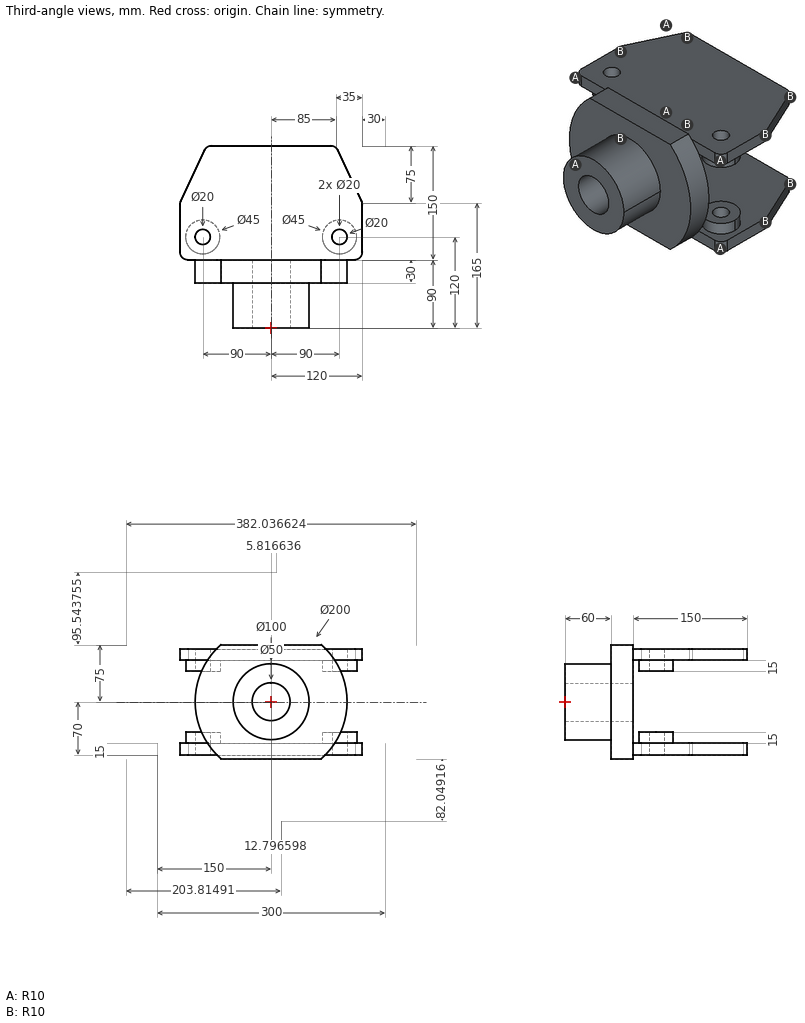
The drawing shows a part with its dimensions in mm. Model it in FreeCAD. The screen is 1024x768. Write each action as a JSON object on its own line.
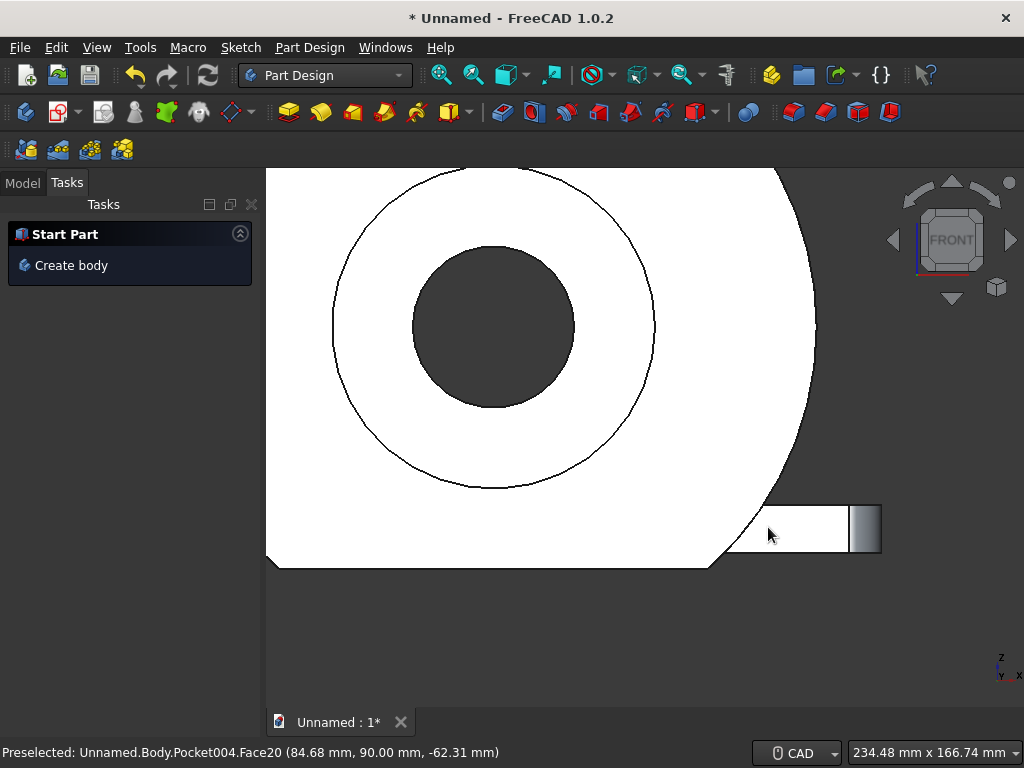
{"action": "left_click", "coordinate": [442, 76]}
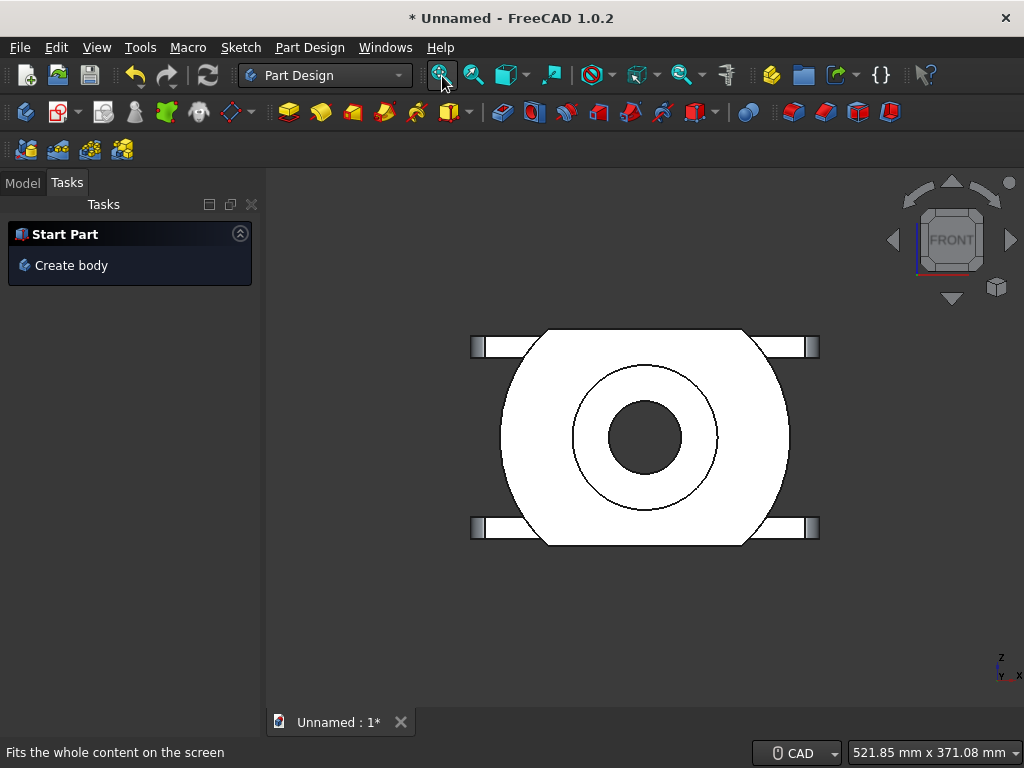
{"action": "key", "text": "3"}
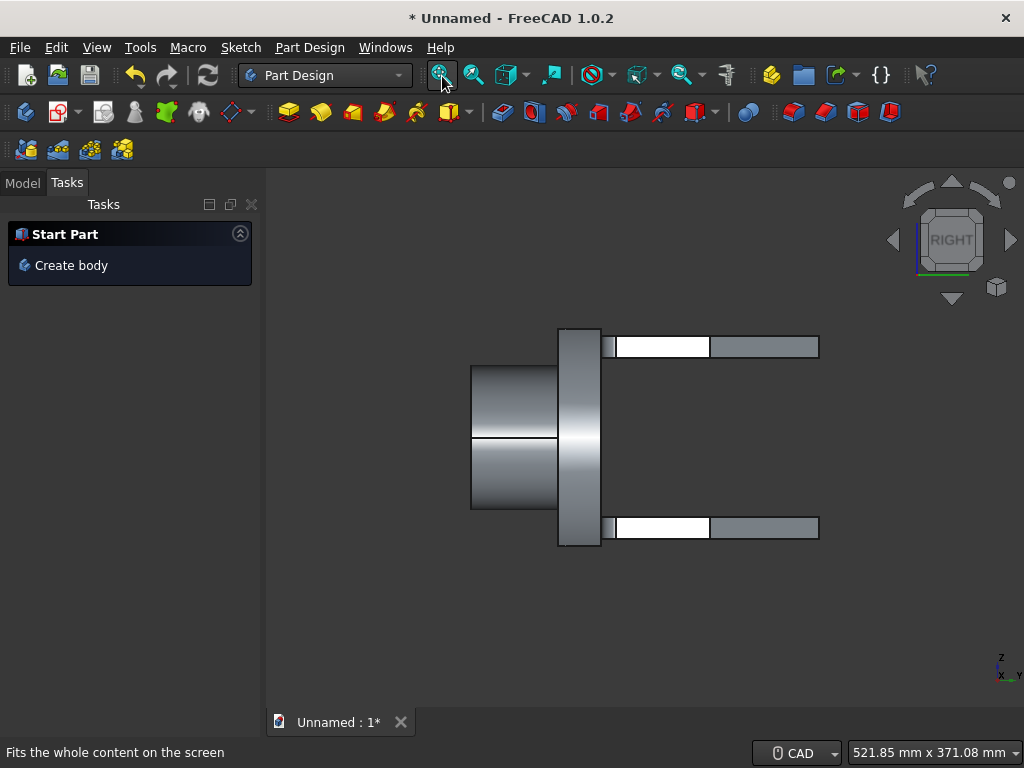
{"action": "left_click", "coordinate": [710, 346]}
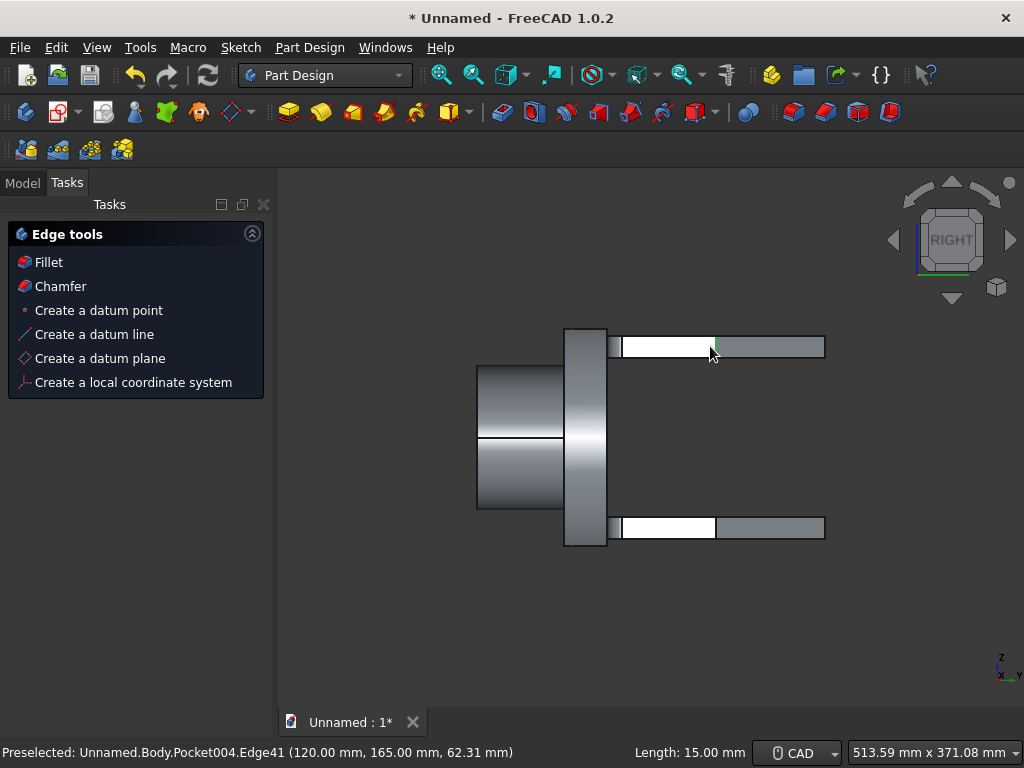
{"action": "left_click", "coordinate": [716, 527], "text": "ctrl"}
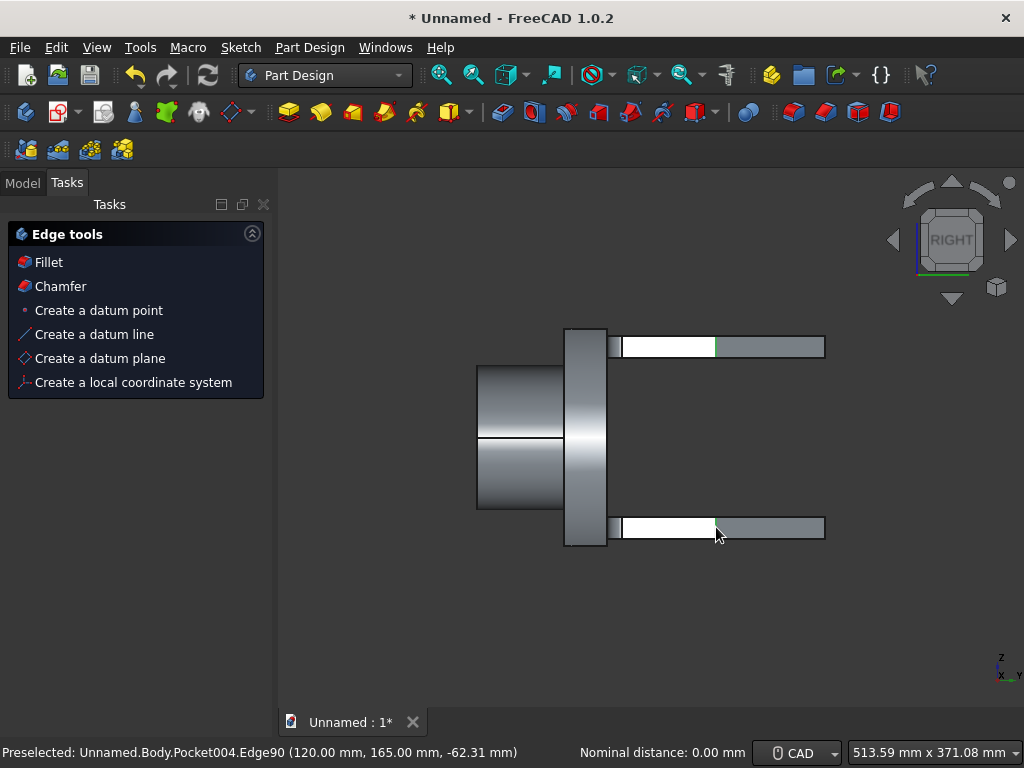
{"action": "scroll", "coordinate": [825, 527], "scroll_direction": "up", "scroll_amount": 4}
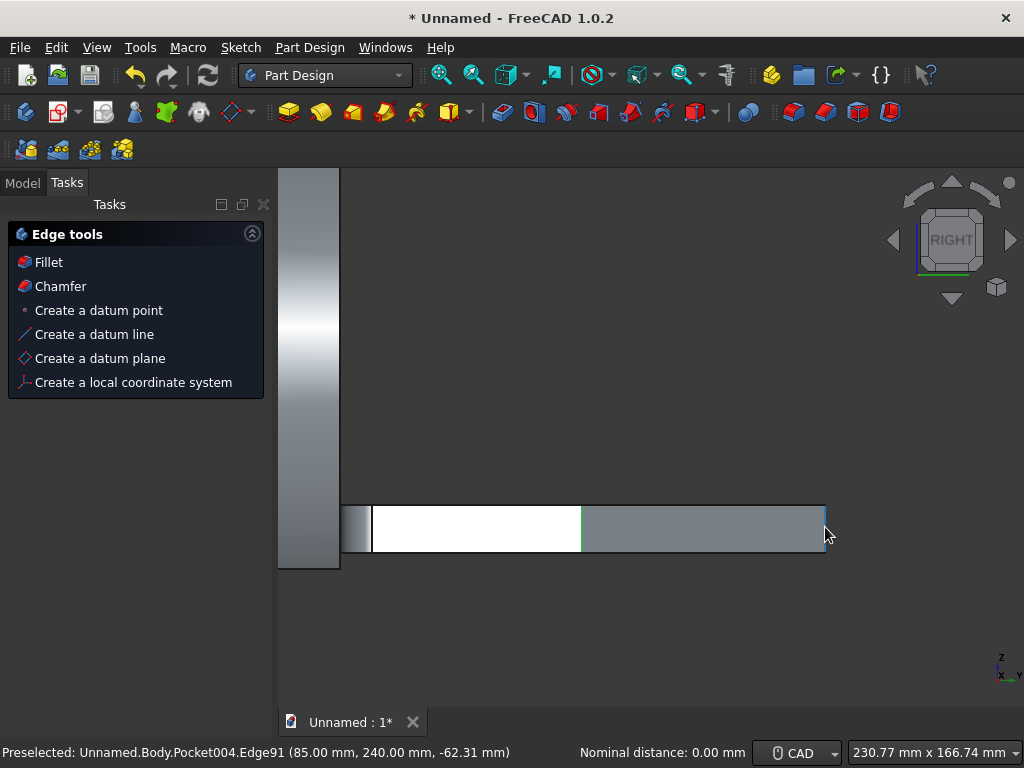
{"action": "left_click", "coordinate": [442, 76]}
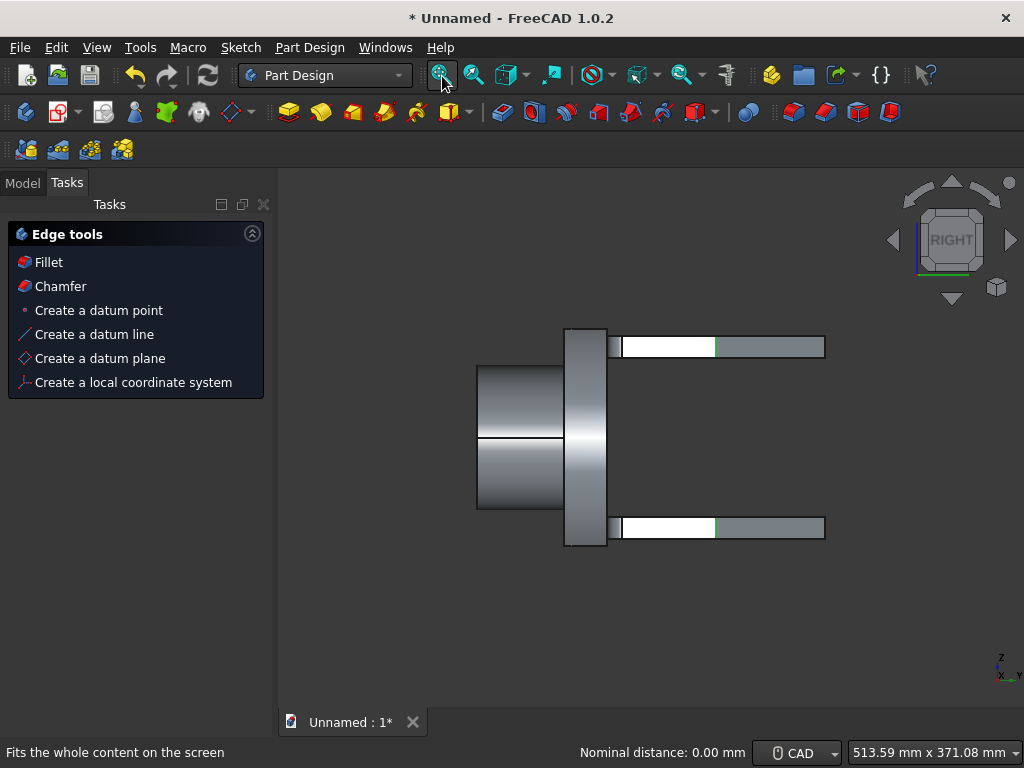
{"action": "key", "text": "5"}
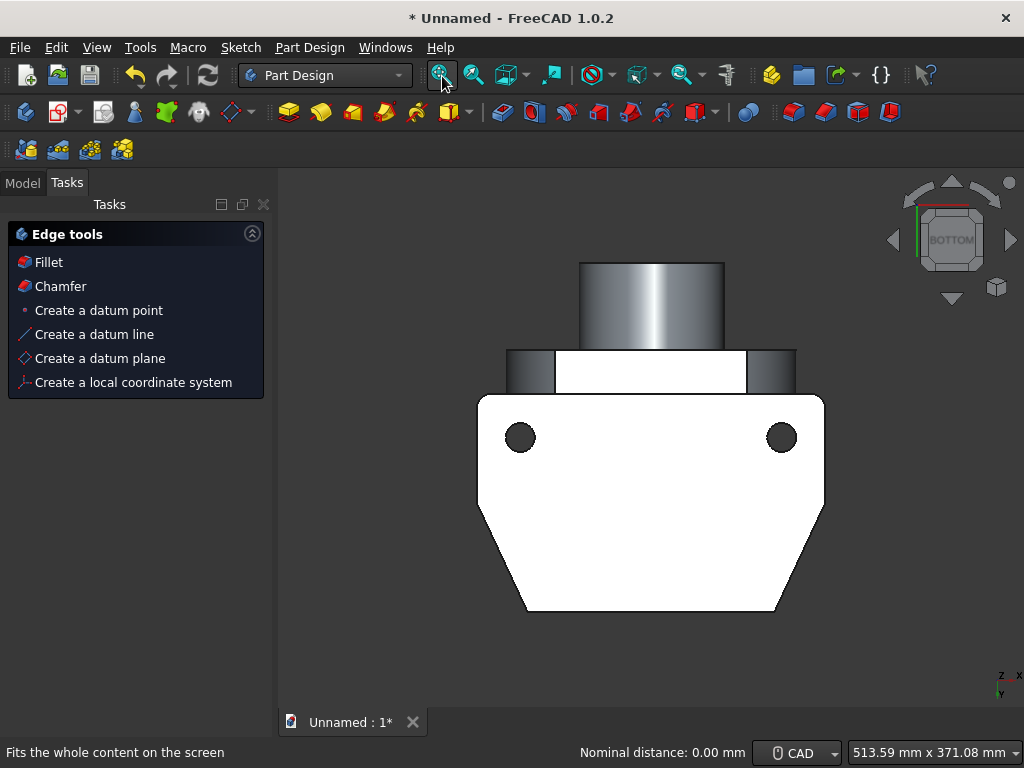
{"action": "scroll", "coordinate": [774, 611], "scroll_direction": "up", "scroll_amount": 4}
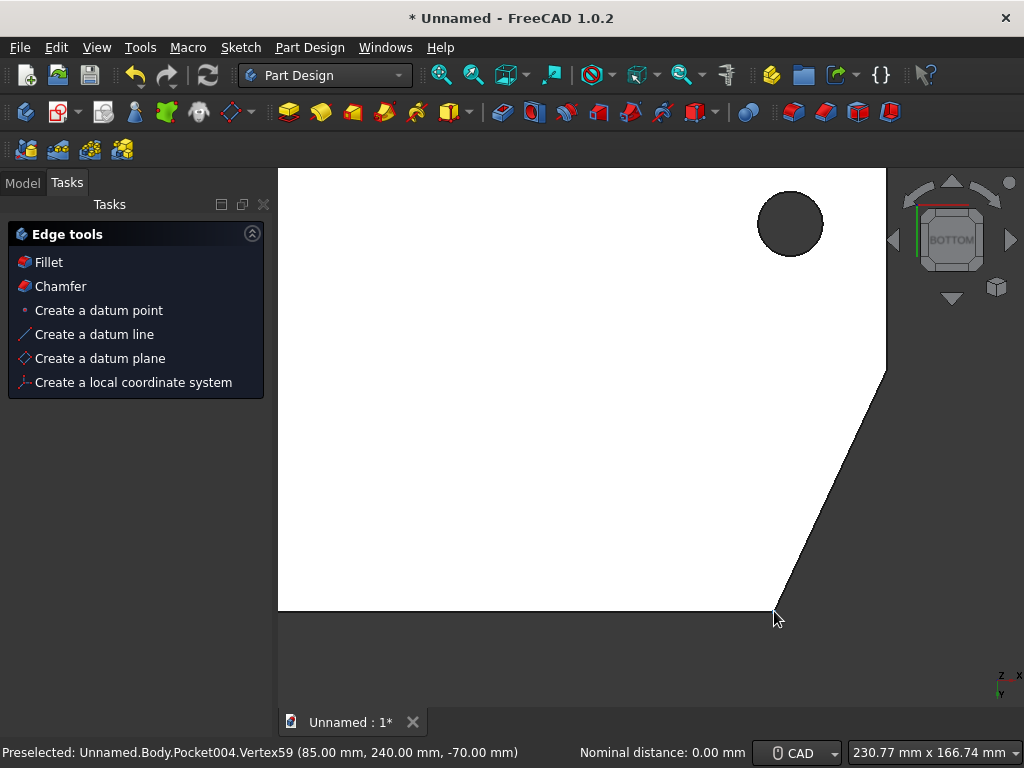
{"action": "left_click", "coordinate": [442, 76]}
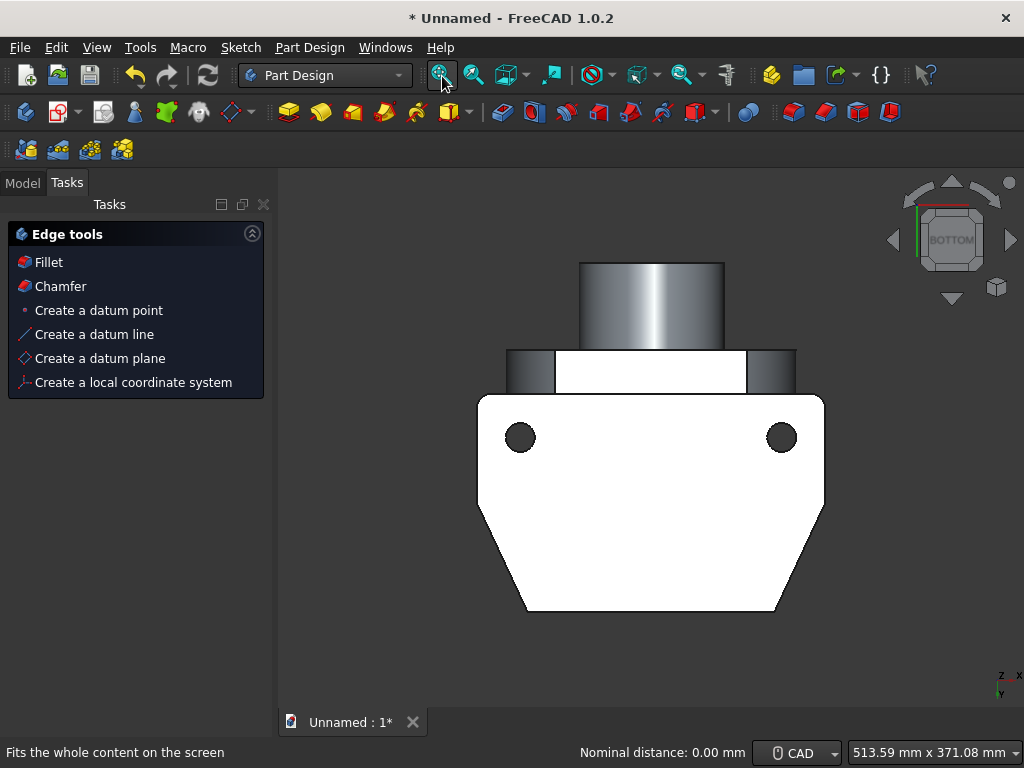
{"action": "key", "text": "4"}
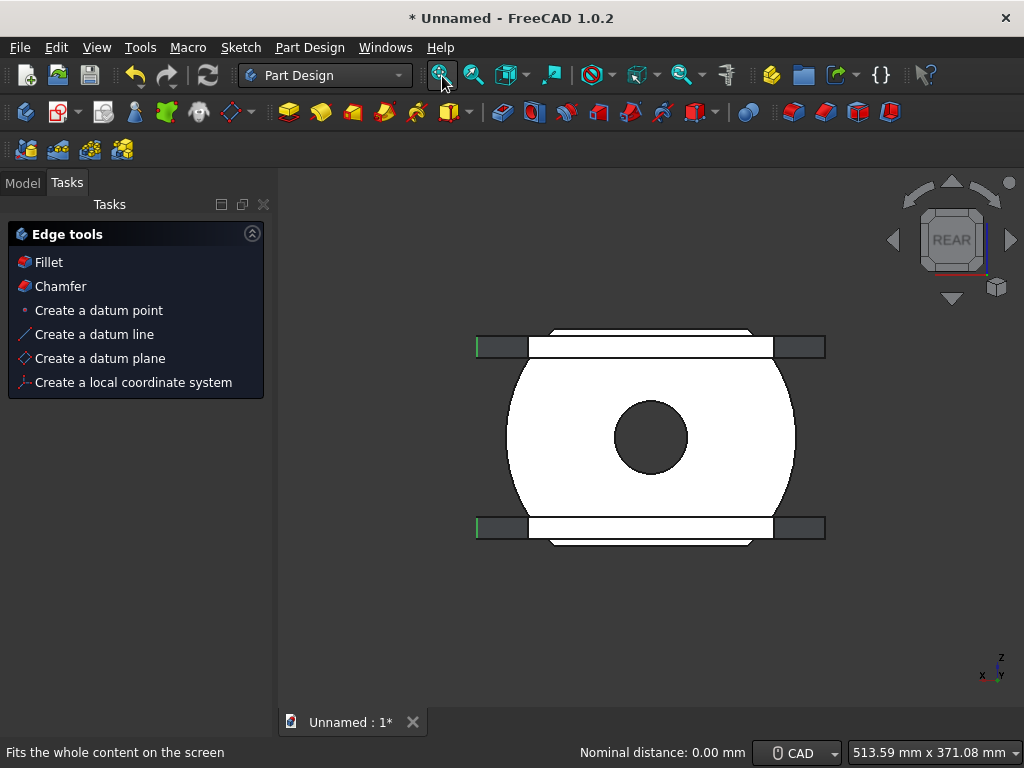
{"action": "left_click", "coordinate": [528, 527], "text": "ctrl"}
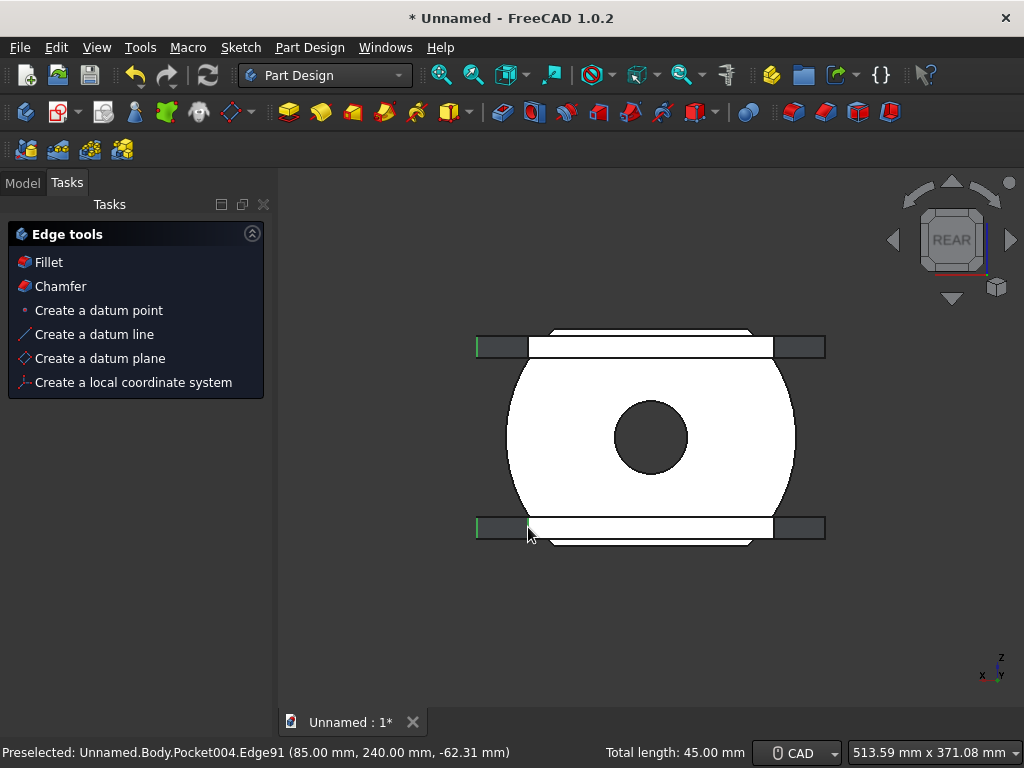
{"action": "left_click", "coordinate": [528, 346], "text": "ctrl"}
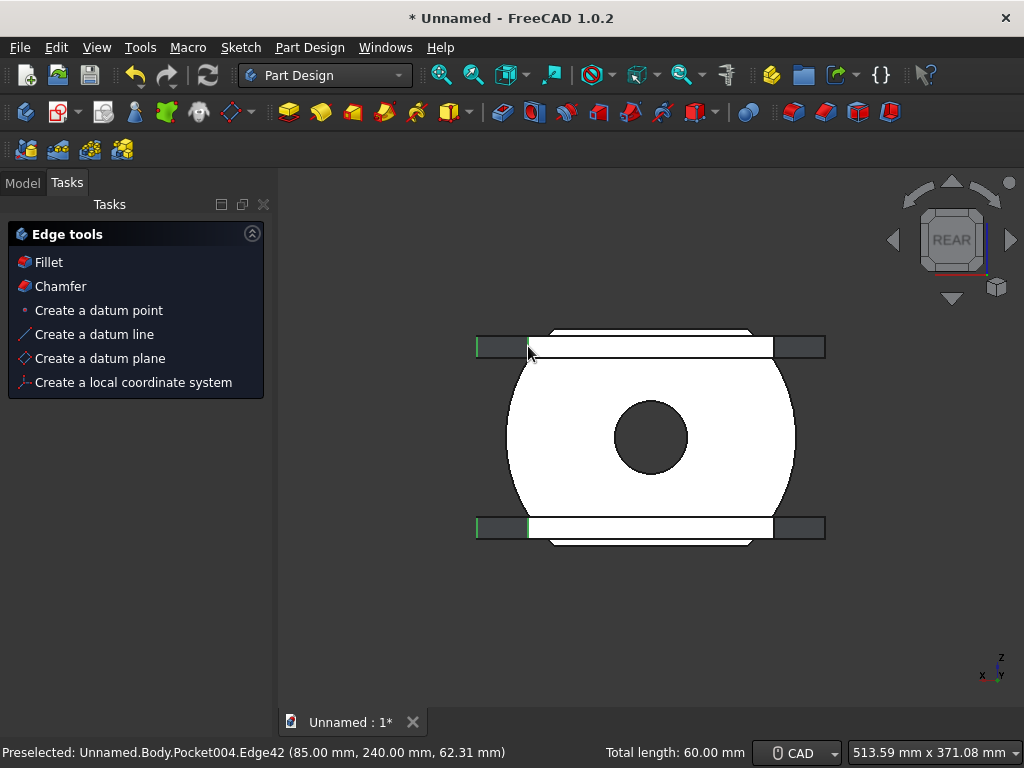
{"action": "left_click", "coordinate": [774, 346], "text": "ctrl"}